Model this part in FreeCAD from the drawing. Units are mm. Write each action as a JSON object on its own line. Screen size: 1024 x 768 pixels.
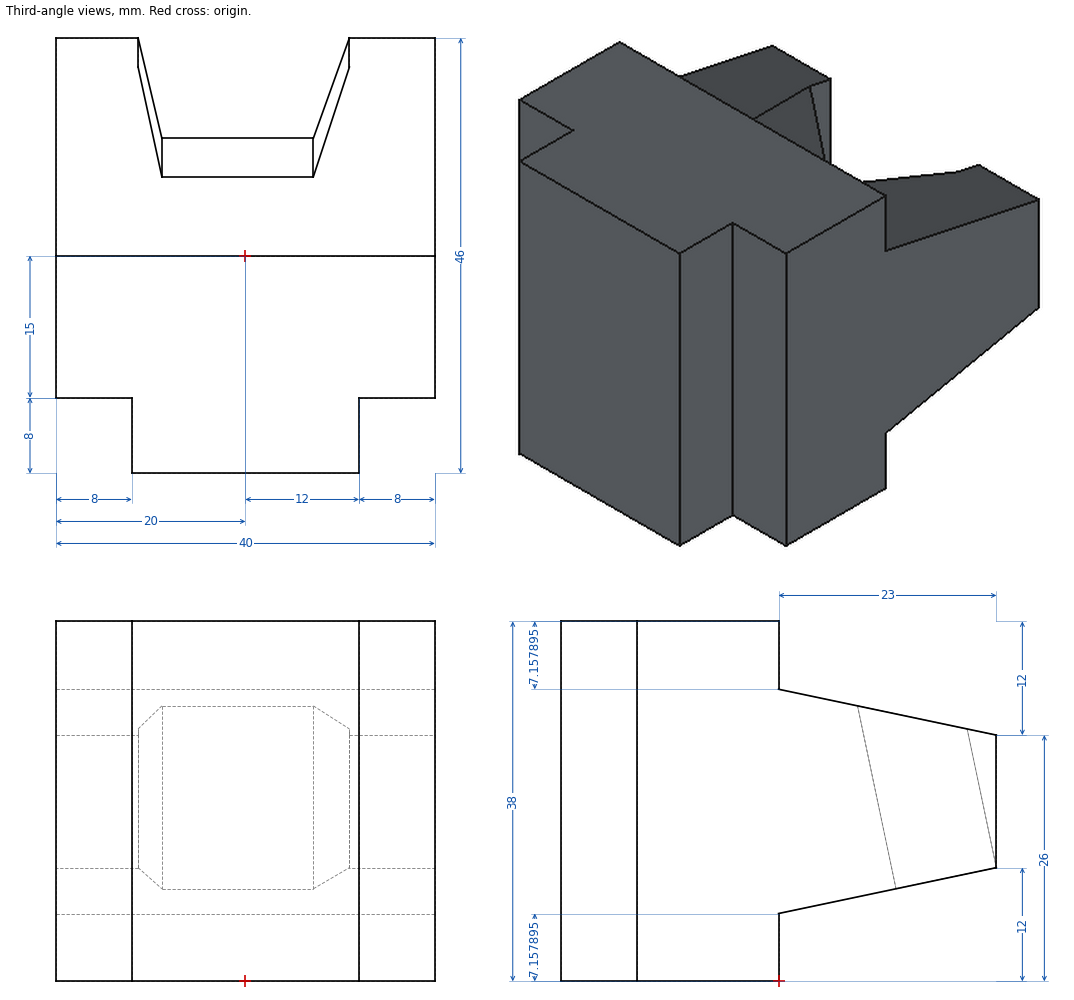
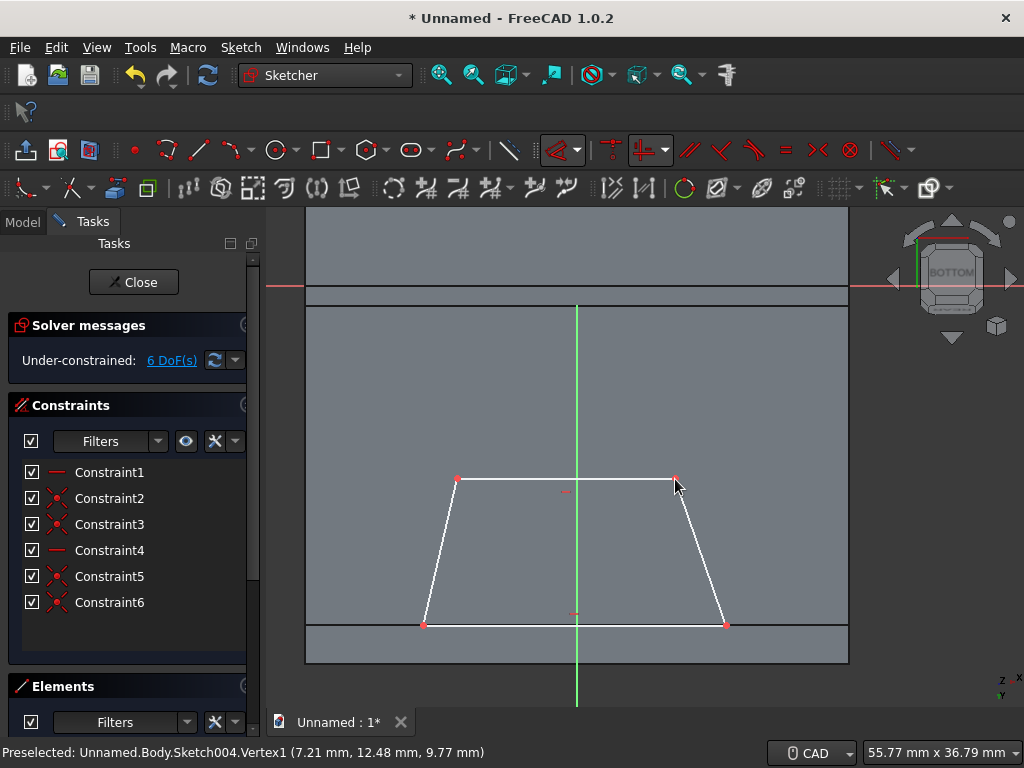
{"action": "left_click", "coordinate": [610, 479]}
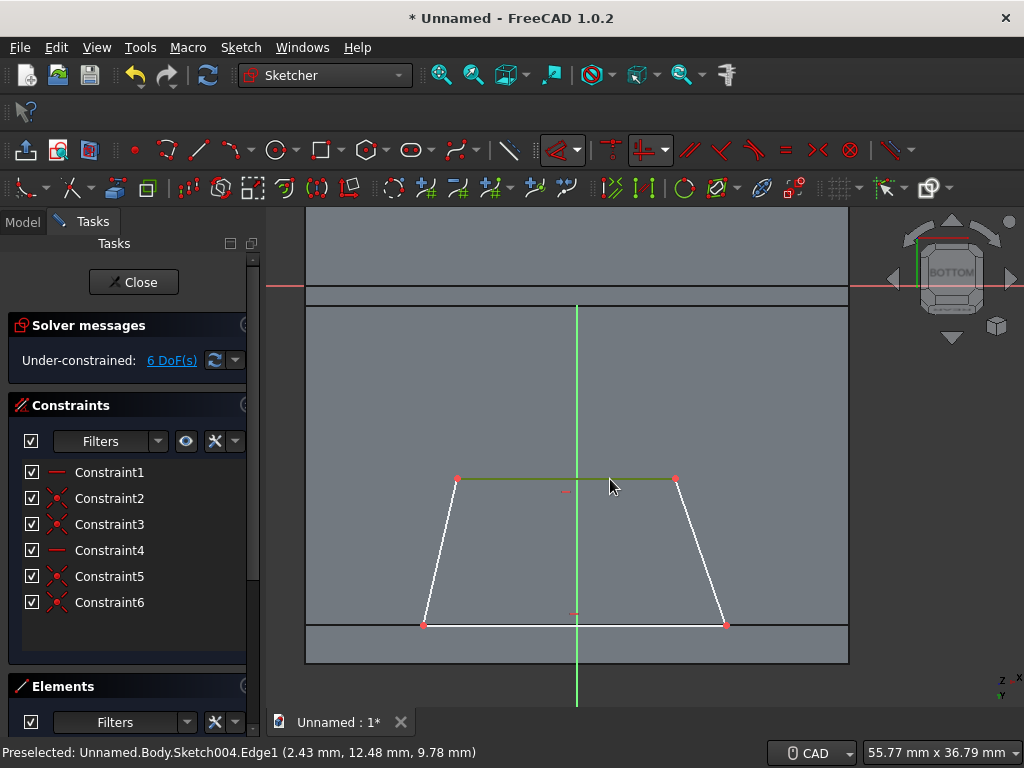
{"action": "key", "text": "l"}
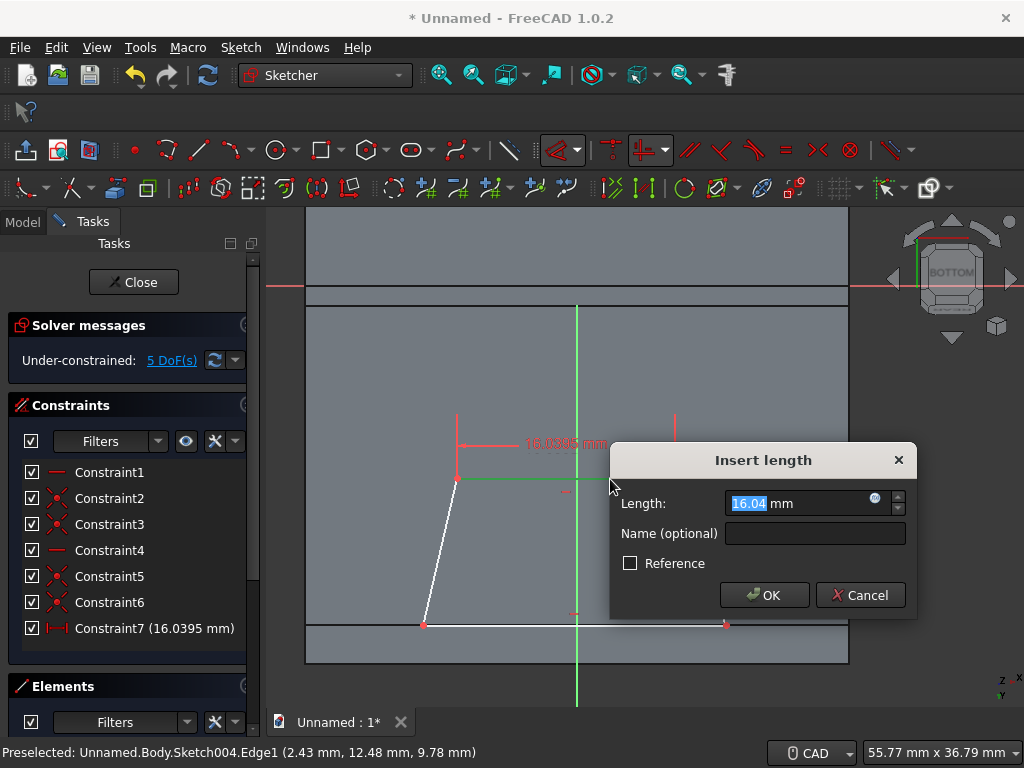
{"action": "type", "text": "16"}
{"action": "key", "text": "Return"}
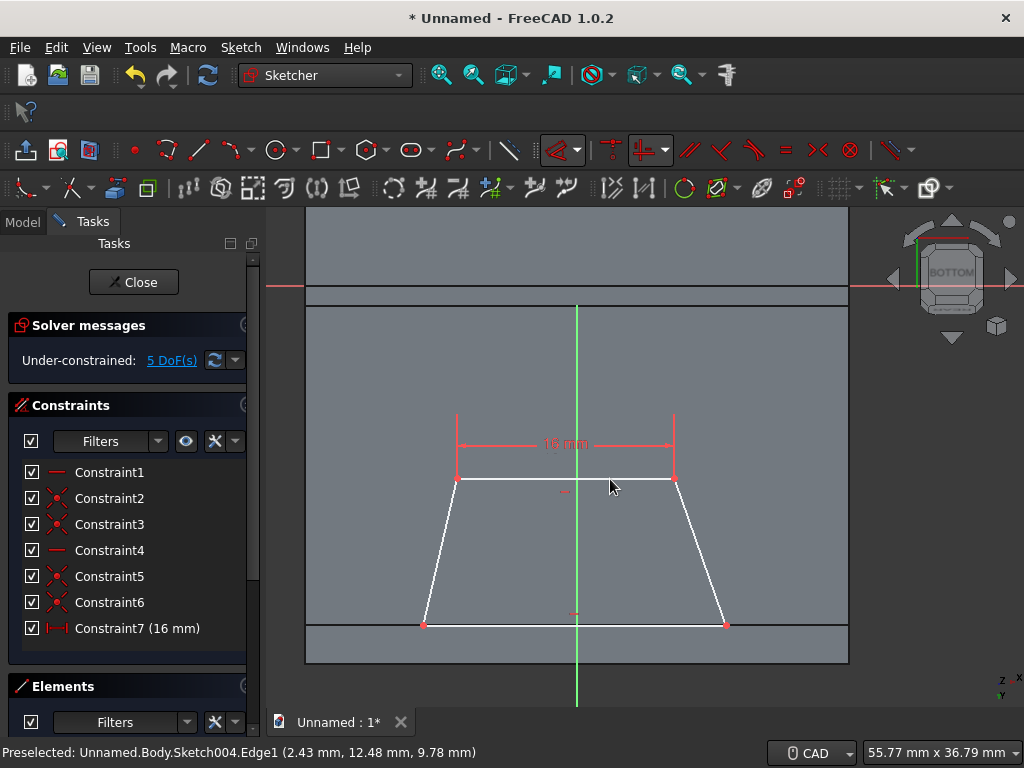
{"action": "left_click", "coordinate": [514, 626]}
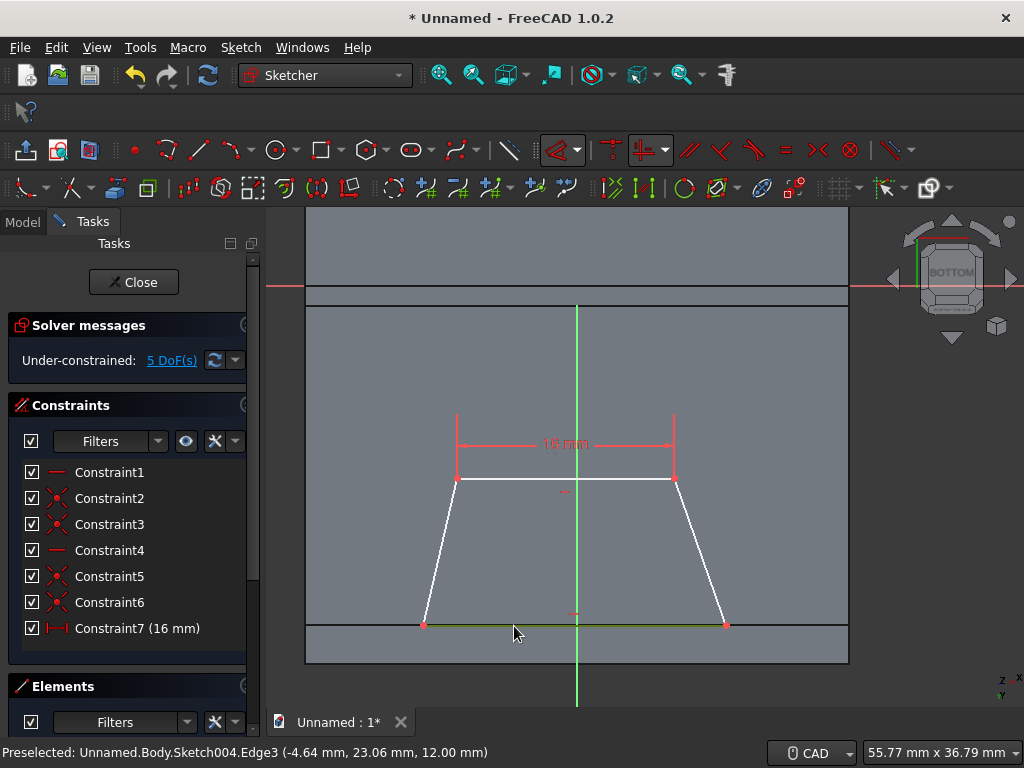
{"action": "key", "text": "l"}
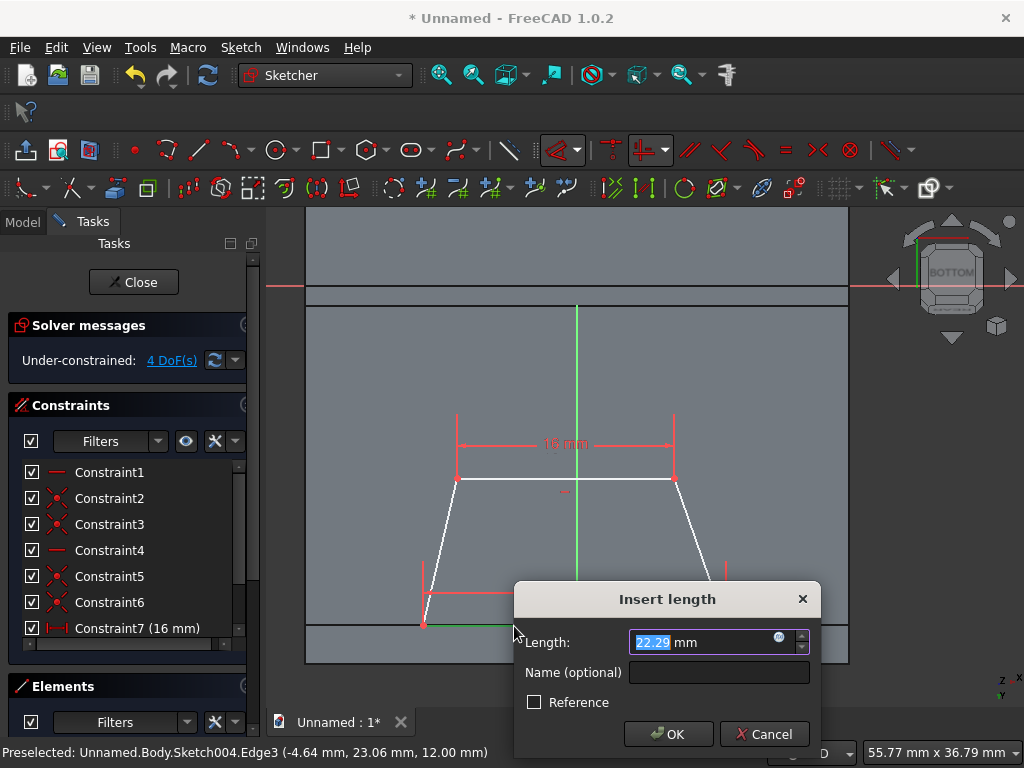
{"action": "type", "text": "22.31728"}
{"action": "key", "text": "Return"}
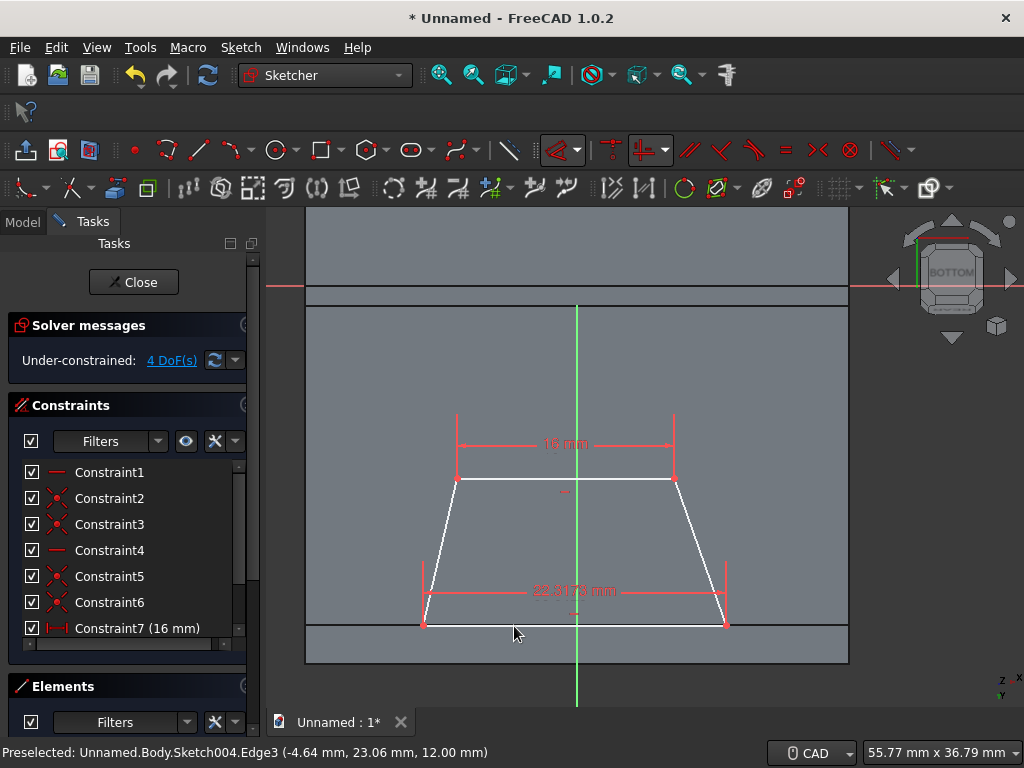
{"action": "left_click", "coordinate": [674, 479]}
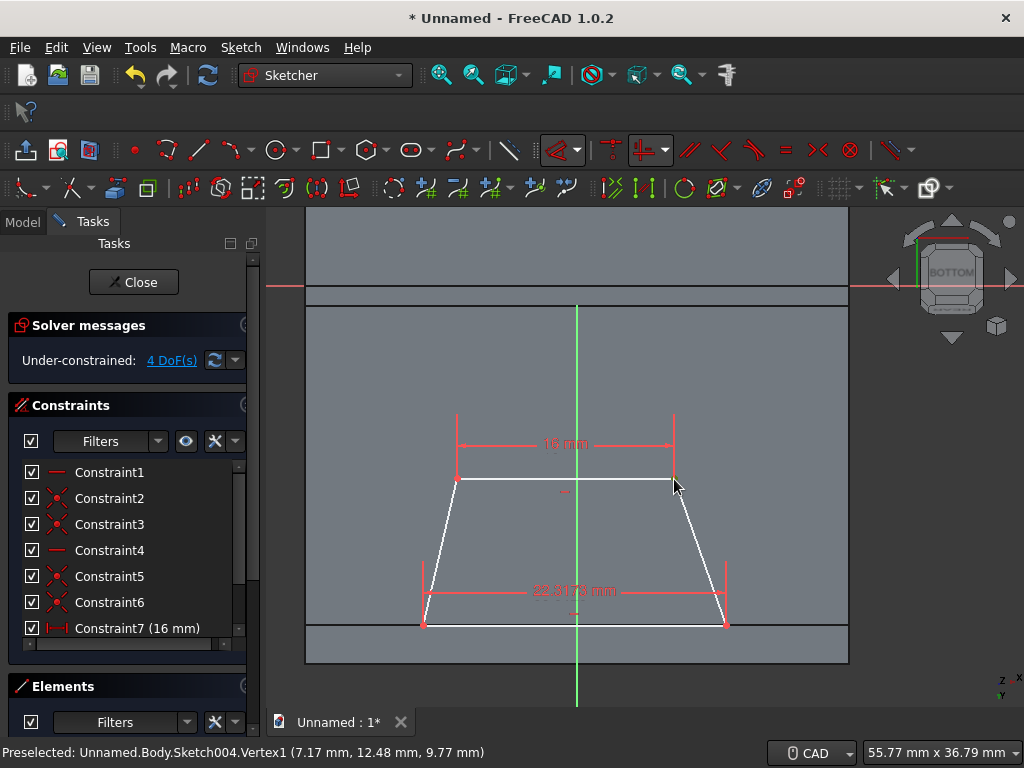
{"action": "left_click", "coordinate": [580, 150]}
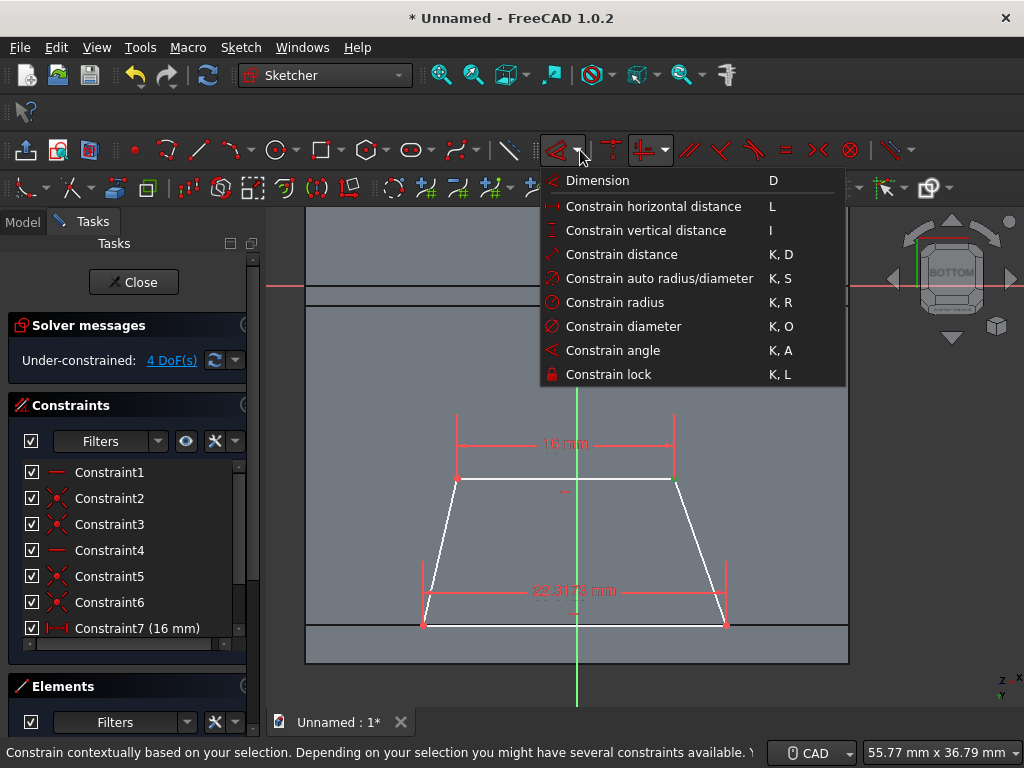
{"action": "left_click", "coordinate": [693, 206]}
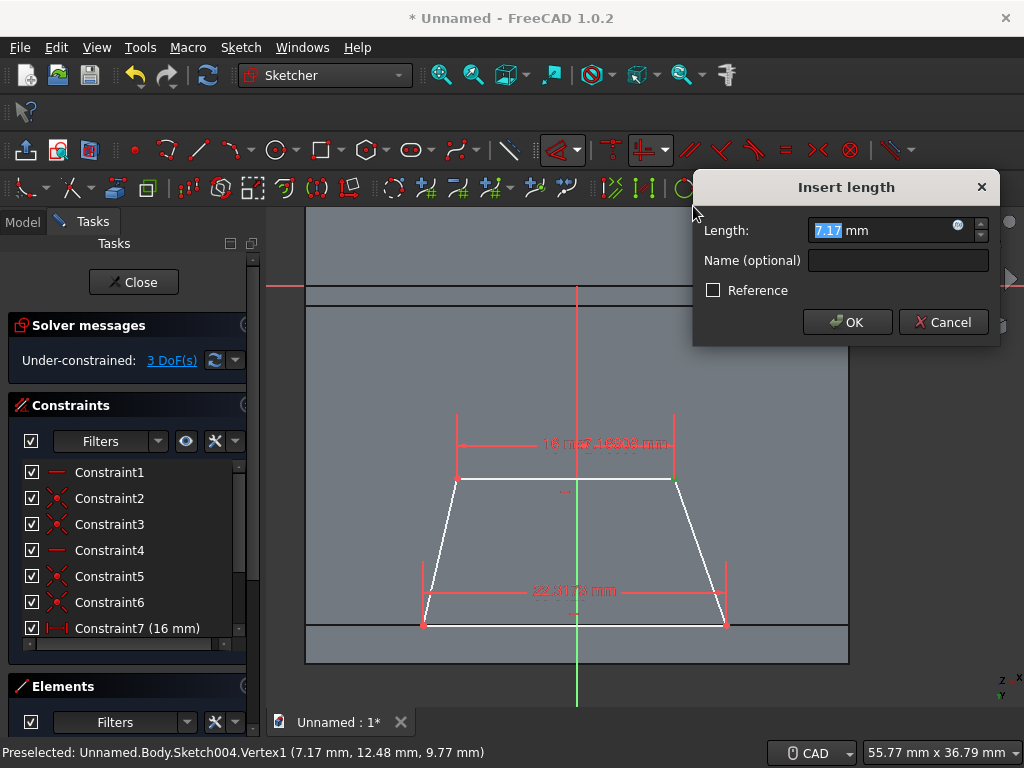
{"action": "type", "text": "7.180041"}
{"action": "key", "text": "Return"}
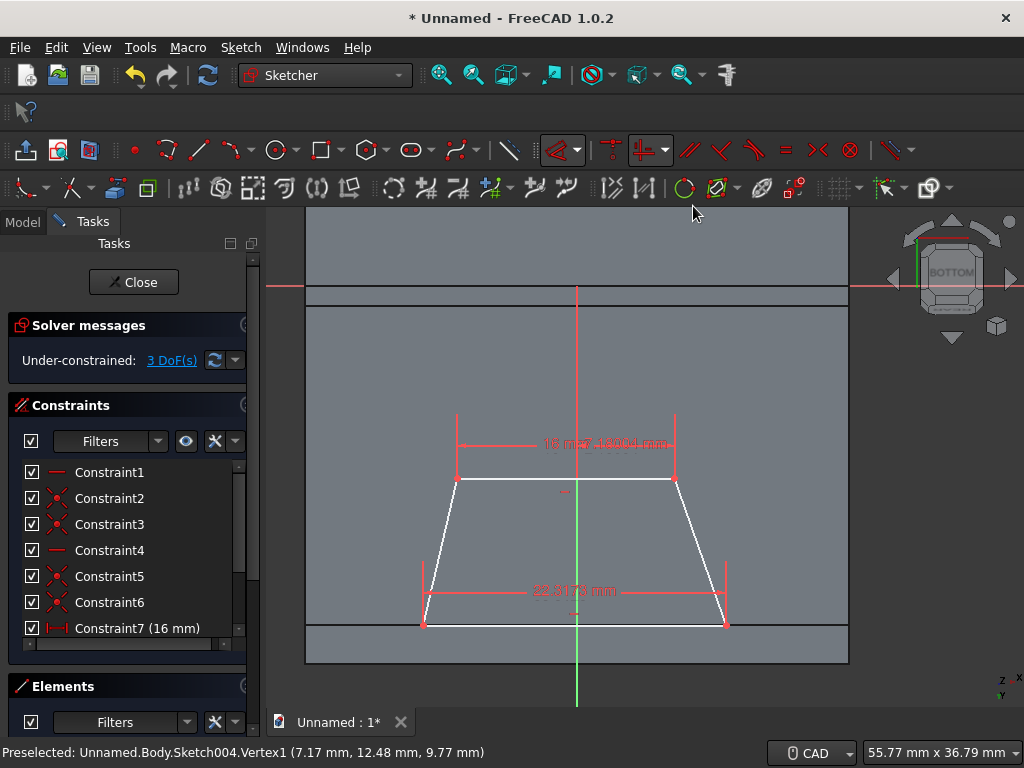
{"action": "left_click", "coordinate": [423, 626]}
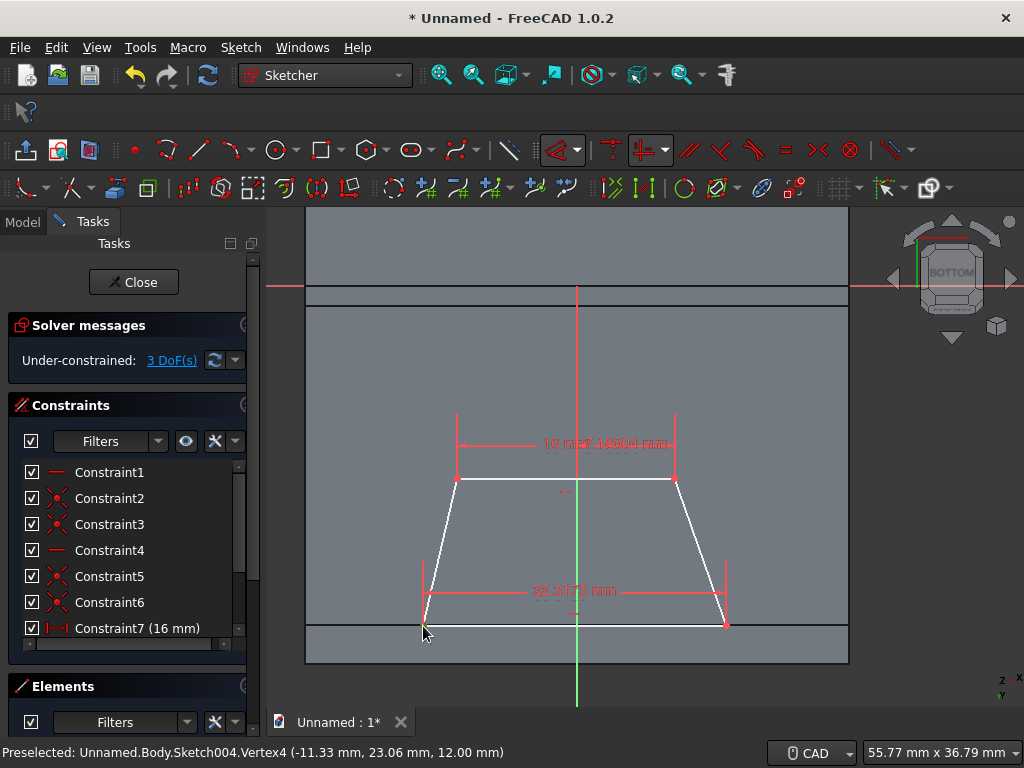
{"action": "left_click", "coordinate": [580, 150]}